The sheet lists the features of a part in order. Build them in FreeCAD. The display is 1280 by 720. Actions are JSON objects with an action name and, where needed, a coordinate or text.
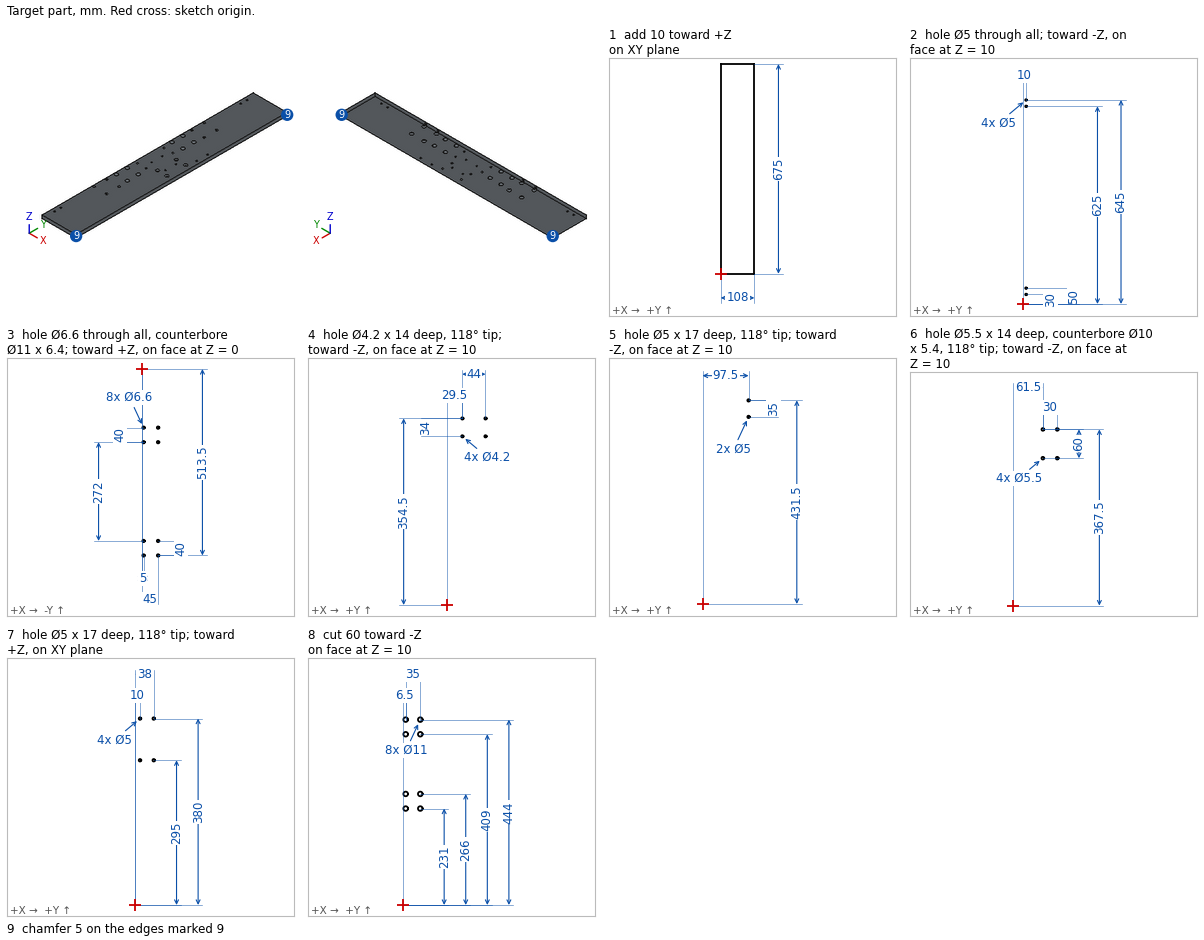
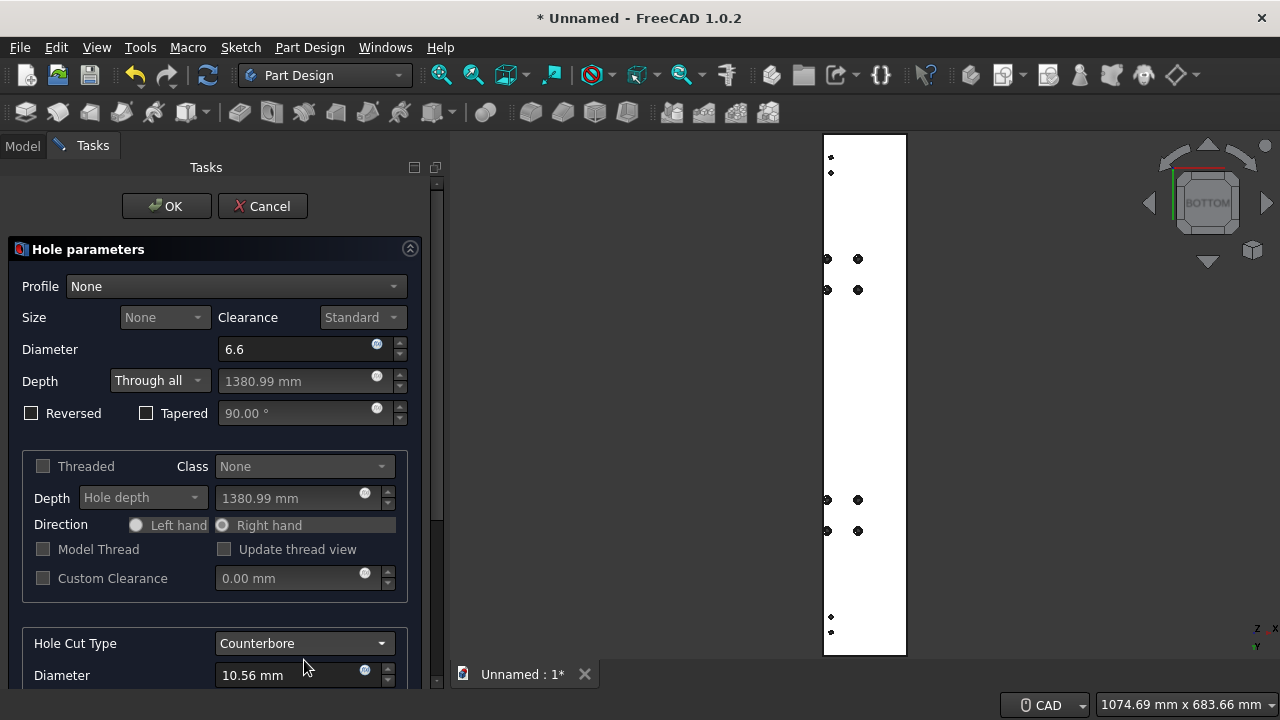
{"action": "triple_click", "coordinate": [298, 675]}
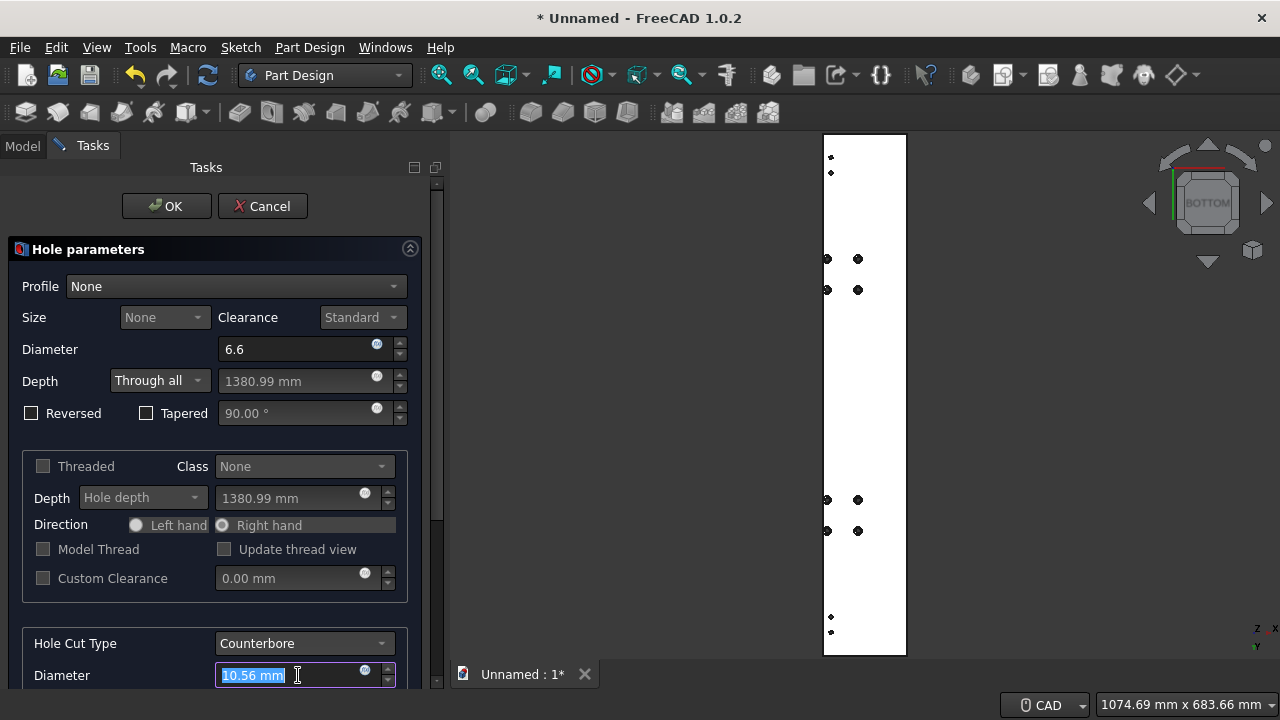
{"action": "type", "text": "11"}
{"action": "key", "text": "Tab"}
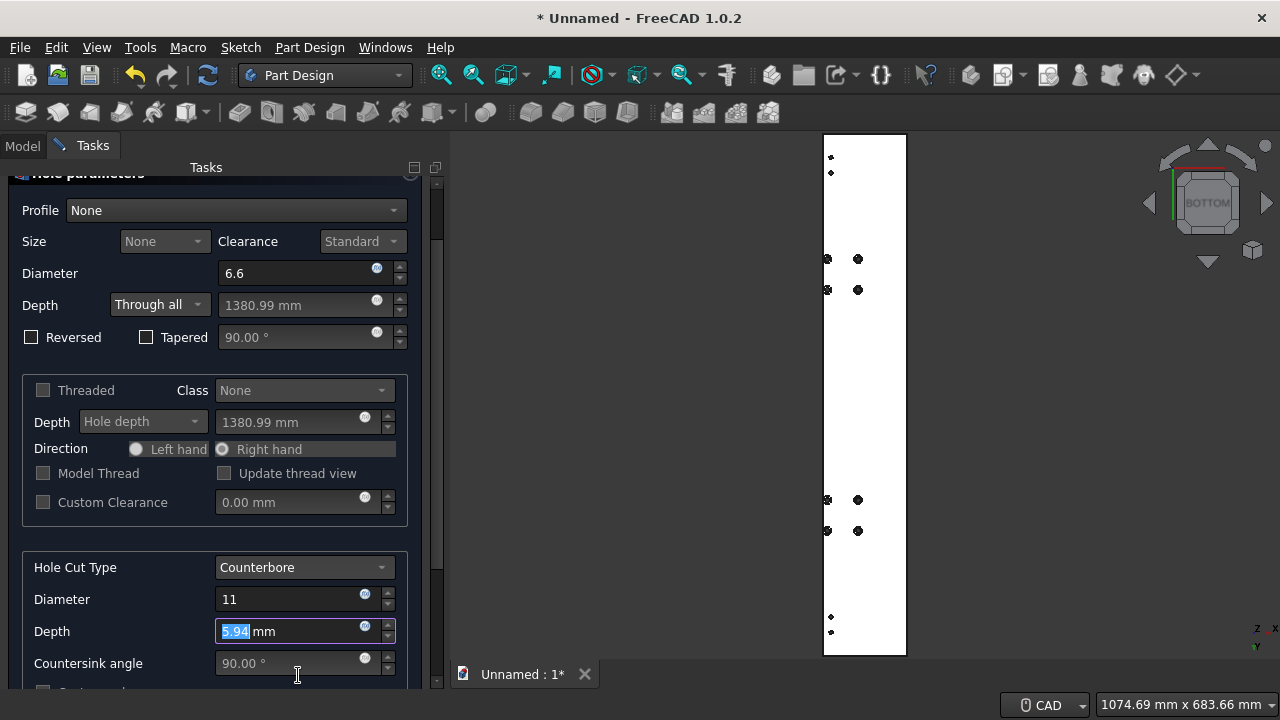
{"action": "type", "text": "6.4"}
{"action": "key", "text": "Tab"}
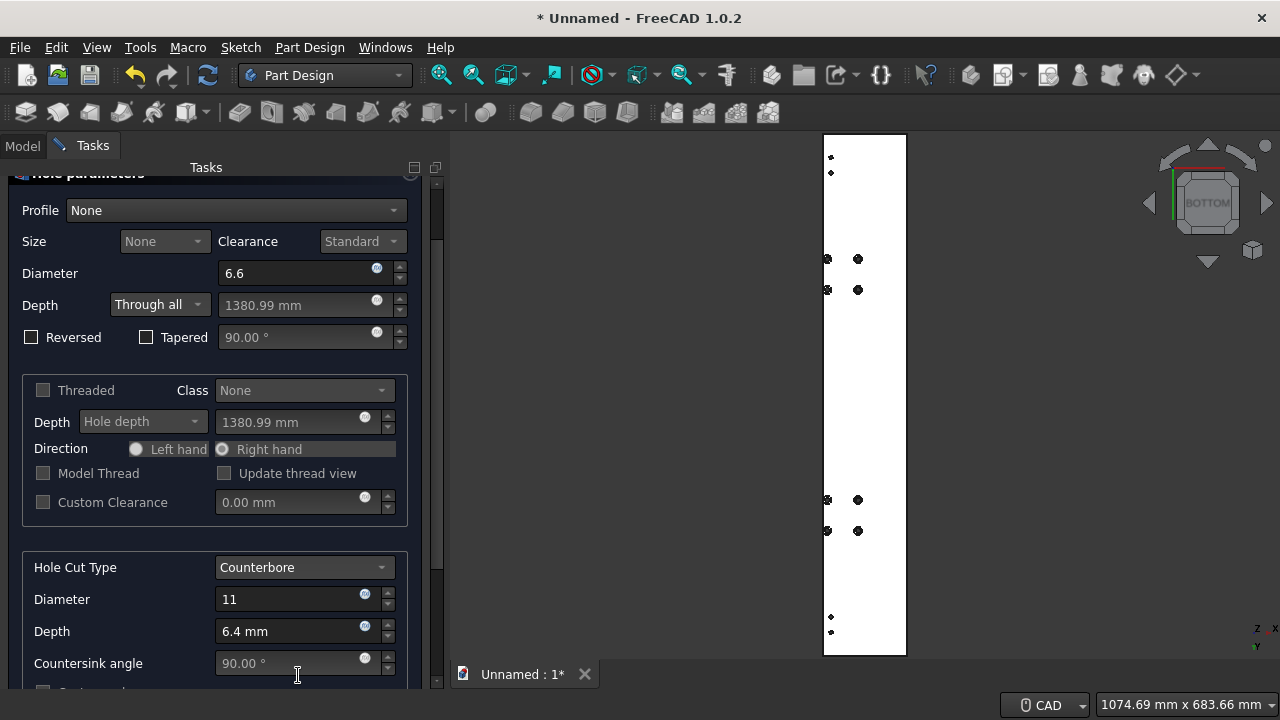
{"action": "scroll", "coordinate": [437, 432], "scroll_direction": "up", "scroll_amount": 3}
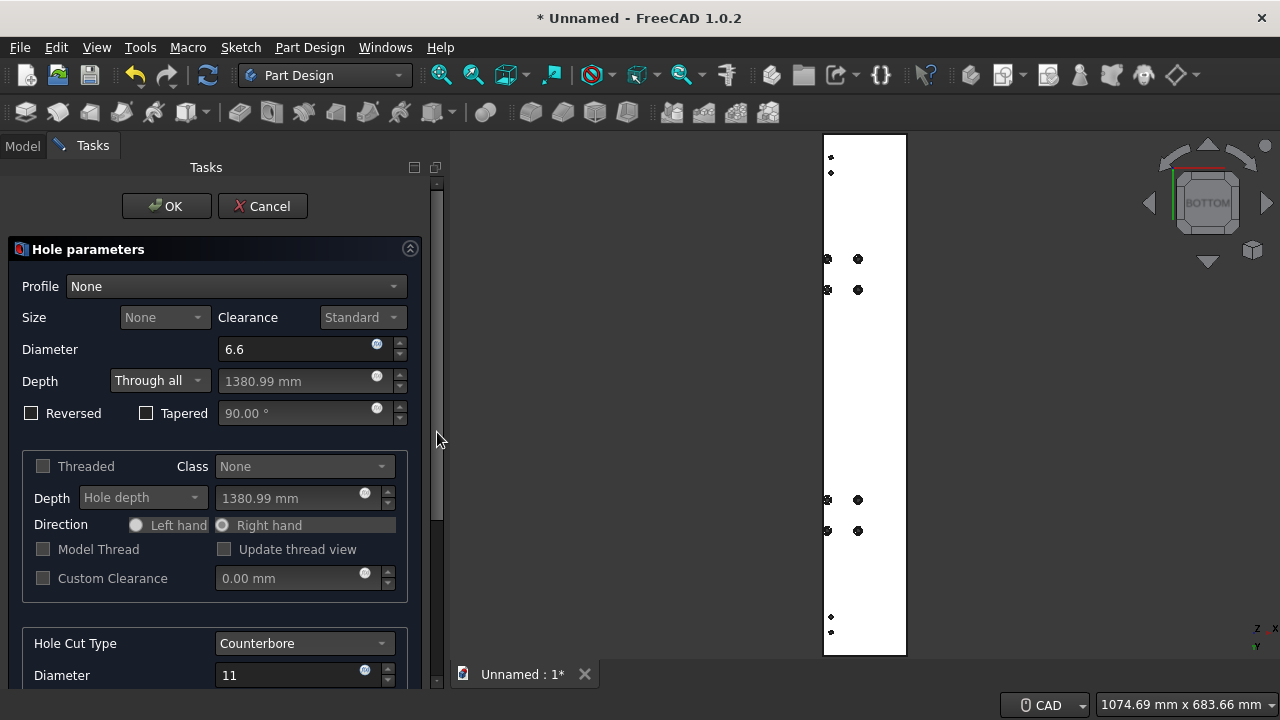
{"action": "left_click", "coordinate": [167, 206]}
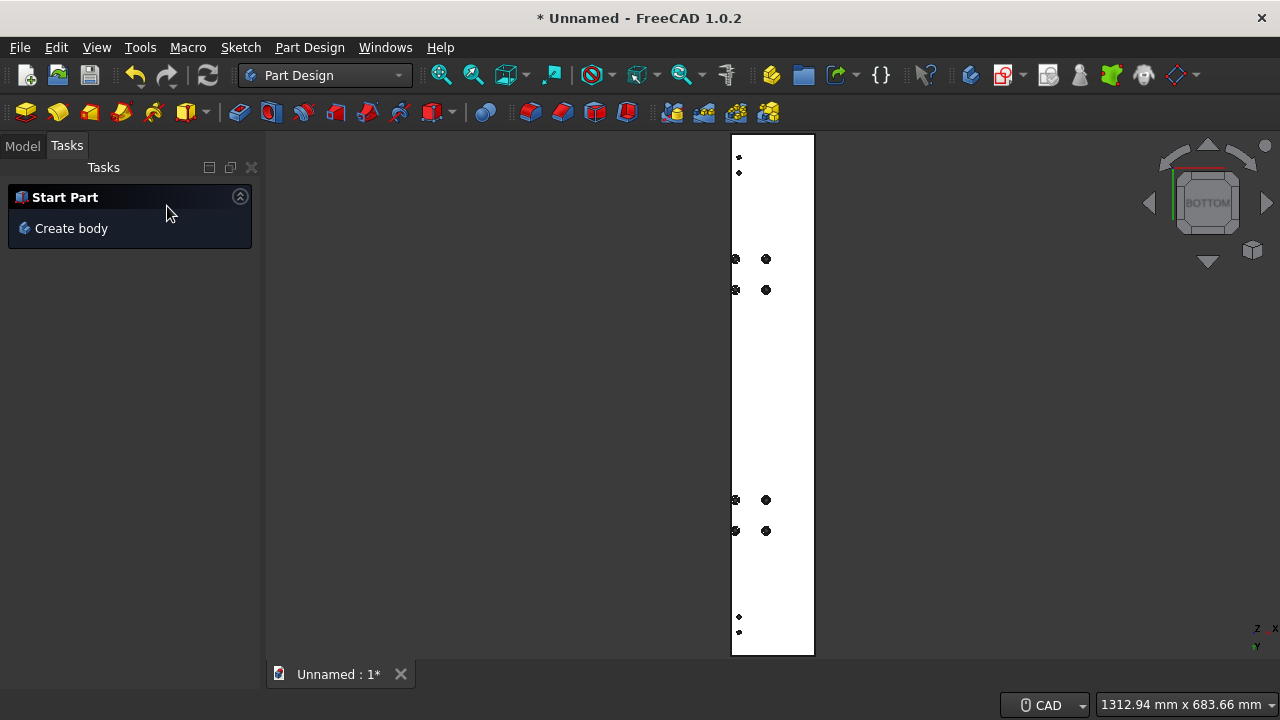
{"action": "key", "text": "0"}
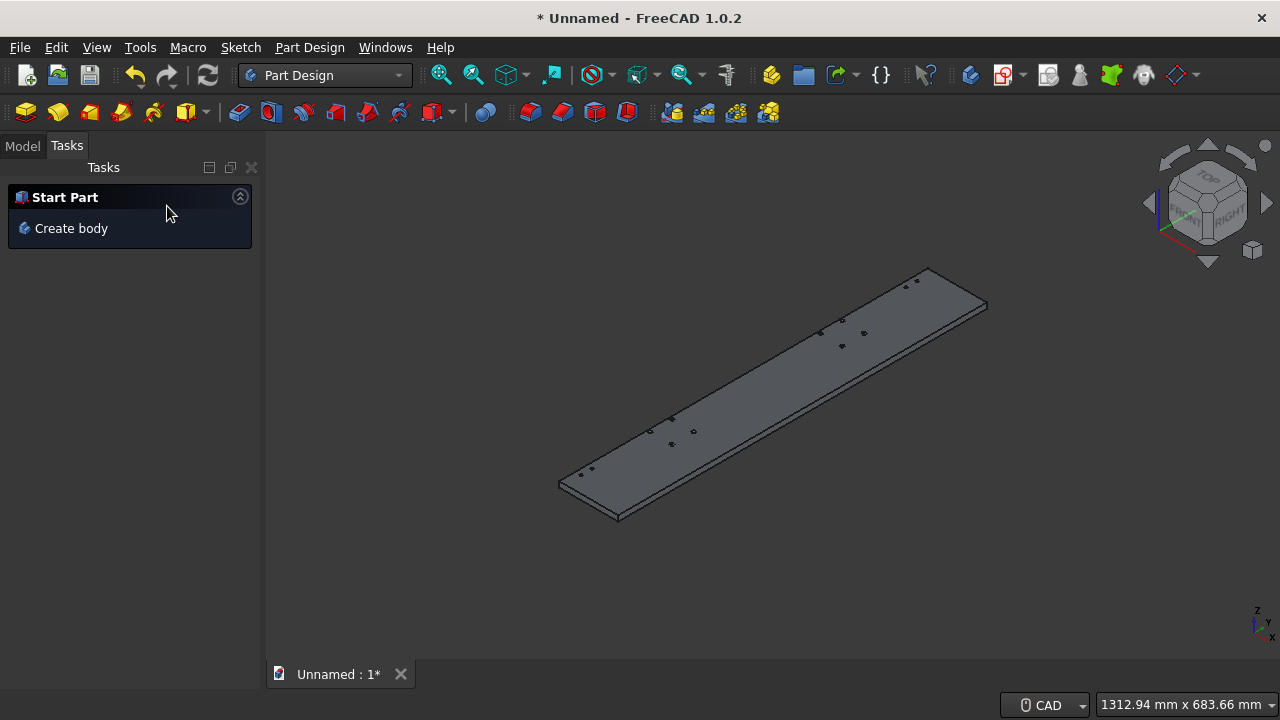
{"action": "left_click", "coordinate": [773, 391]}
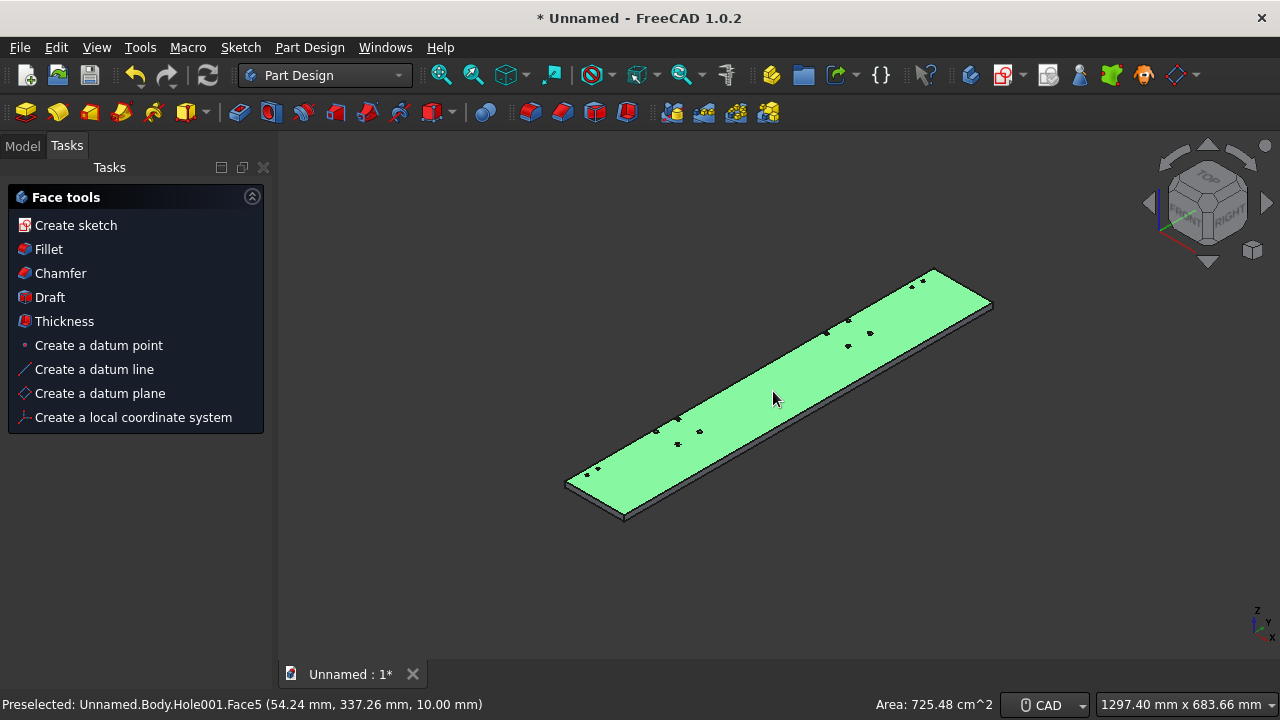
{"action": "left_click", "coordinate": [1004, 76]}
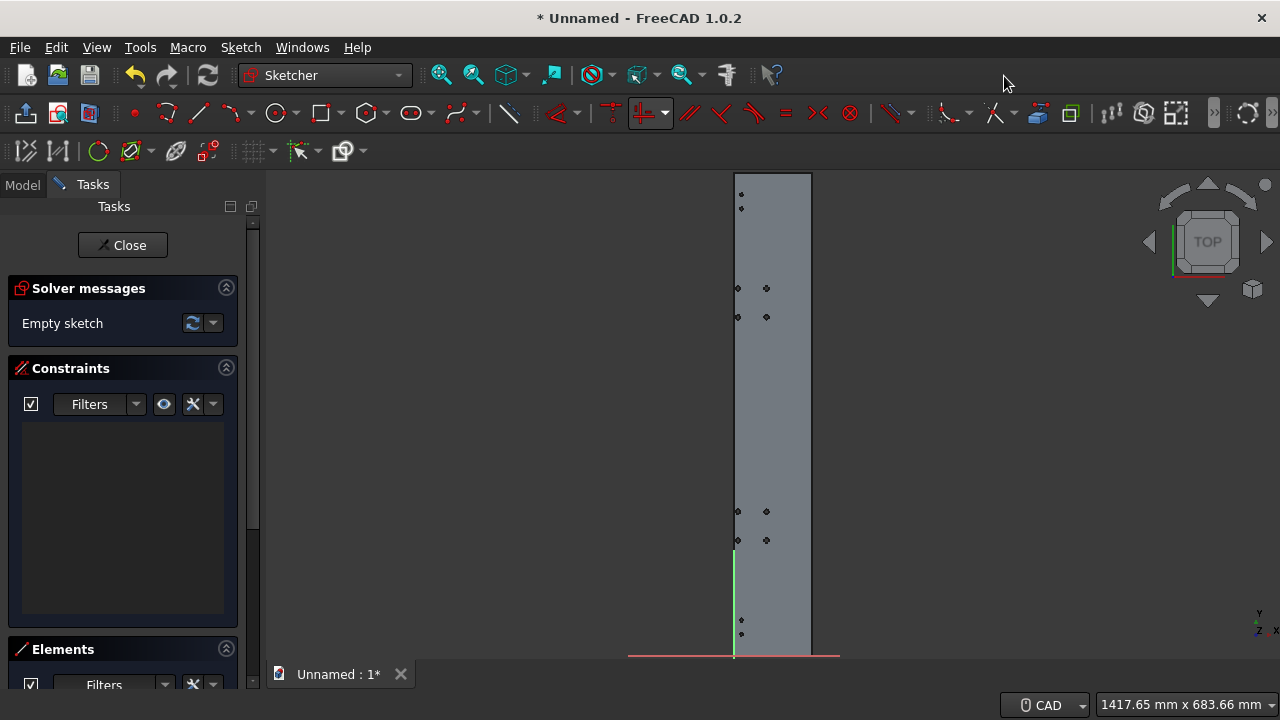
{"action": "scroll", "coordinate": [778, 415], "scroll_direction": "up", "scroll_amount": 12}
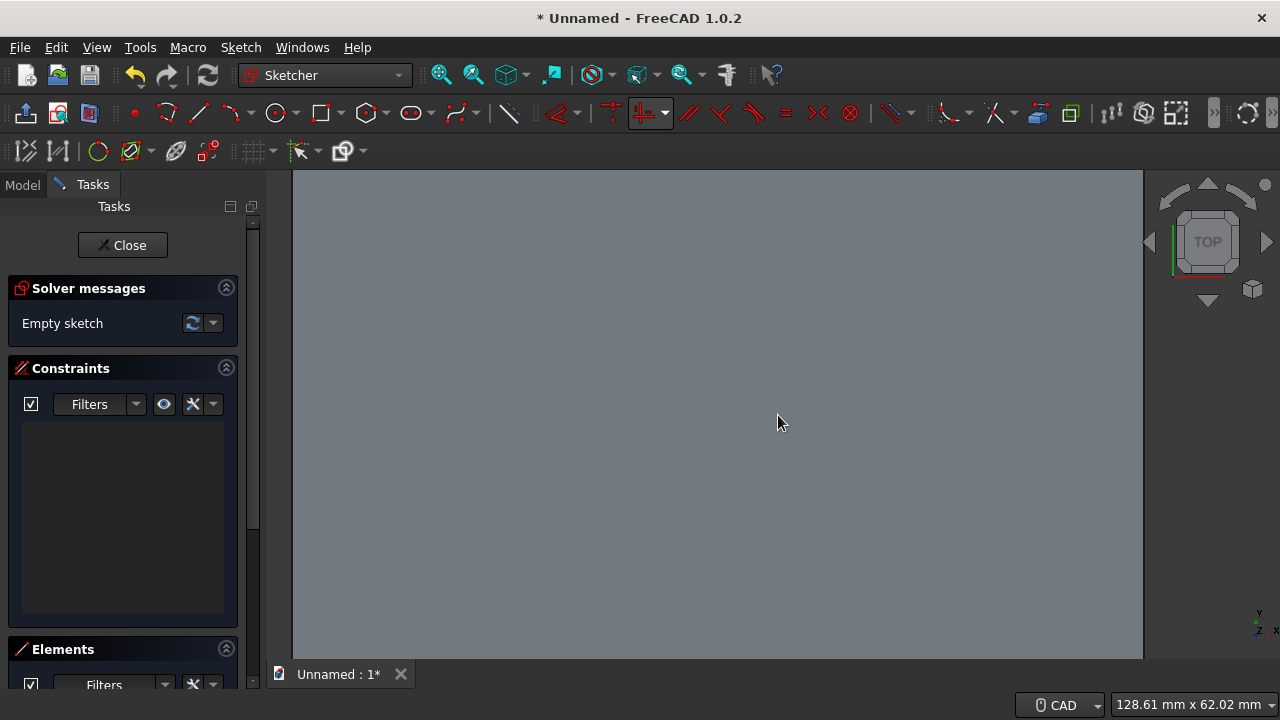
{"action": "left_click", "coordinate": [276, 114]}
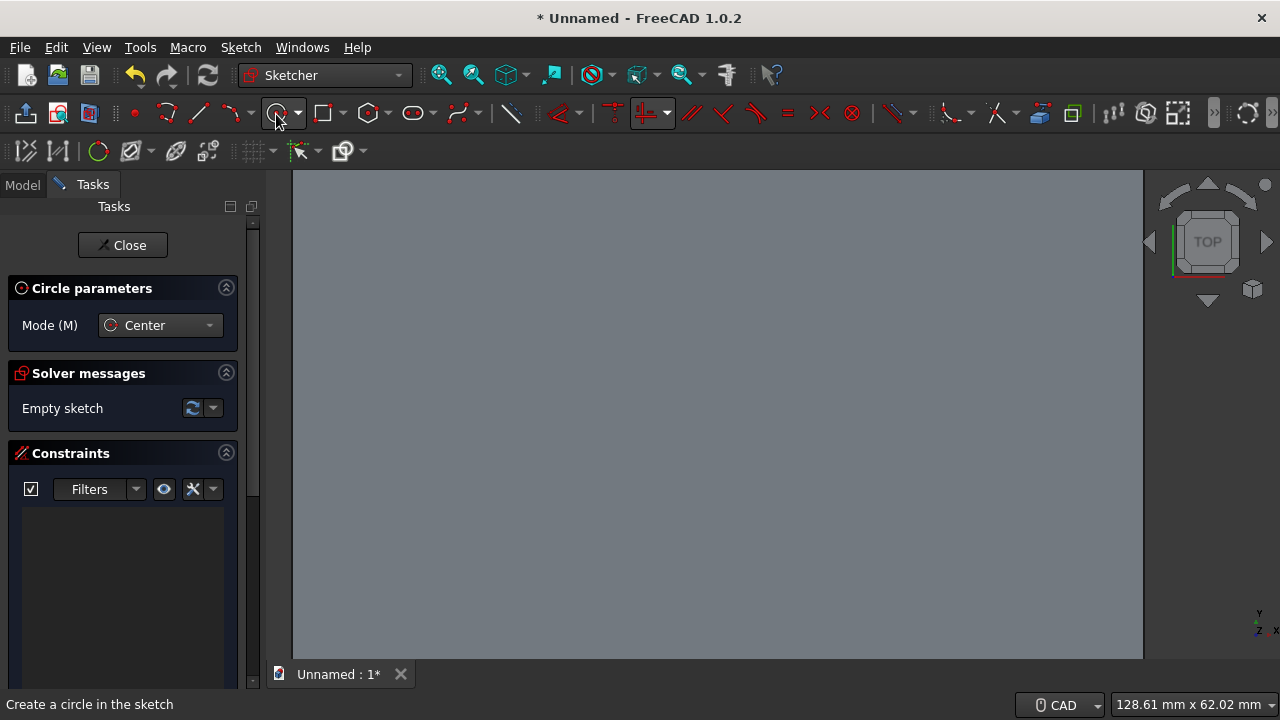
{"action": "scroll", "coordinate": [525, 270], "scroll_direction": "up", "scroll_amount": 2}